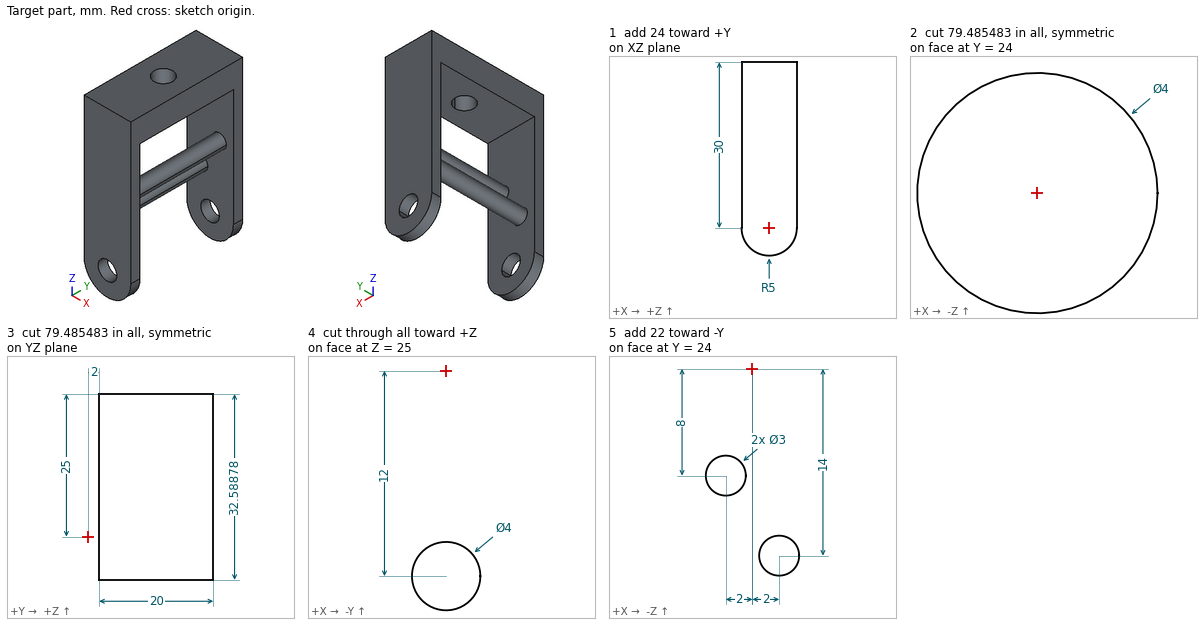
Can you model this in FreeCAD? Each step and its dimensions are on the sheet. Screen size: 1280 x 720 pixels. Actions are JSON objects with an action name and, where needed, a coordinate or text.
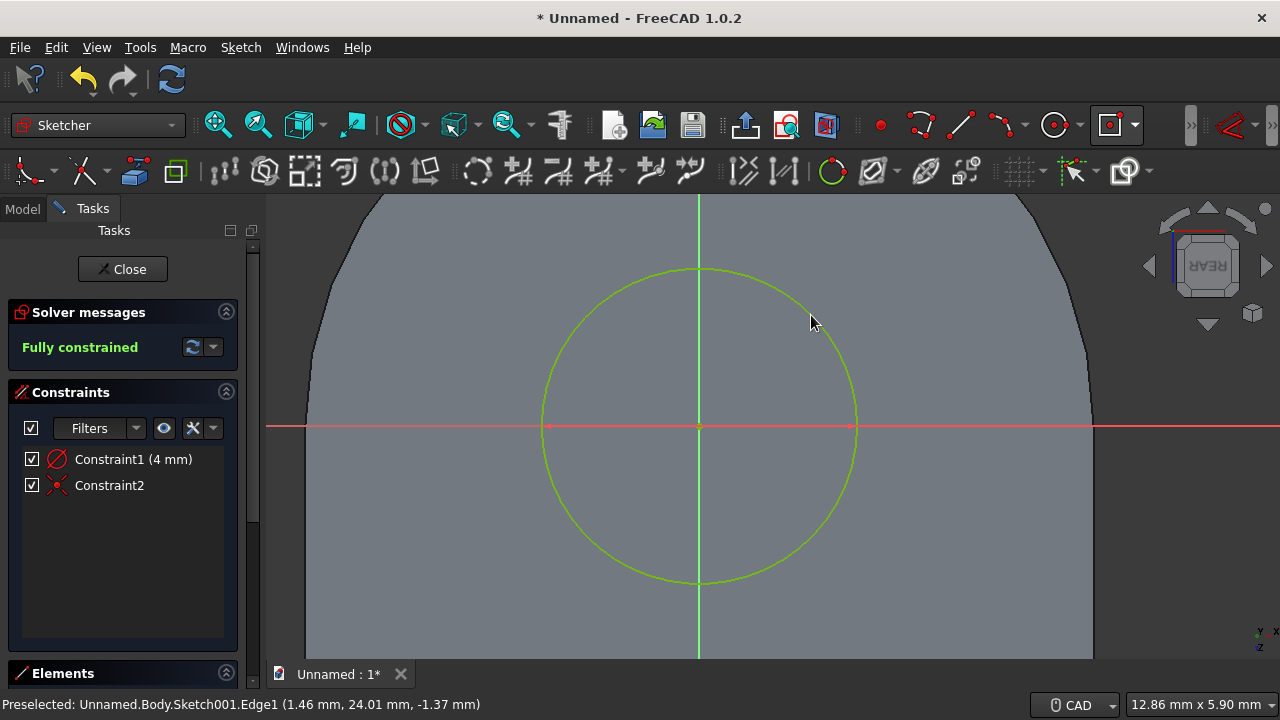
{"action": "left_click", "coordinate": [123, 269]}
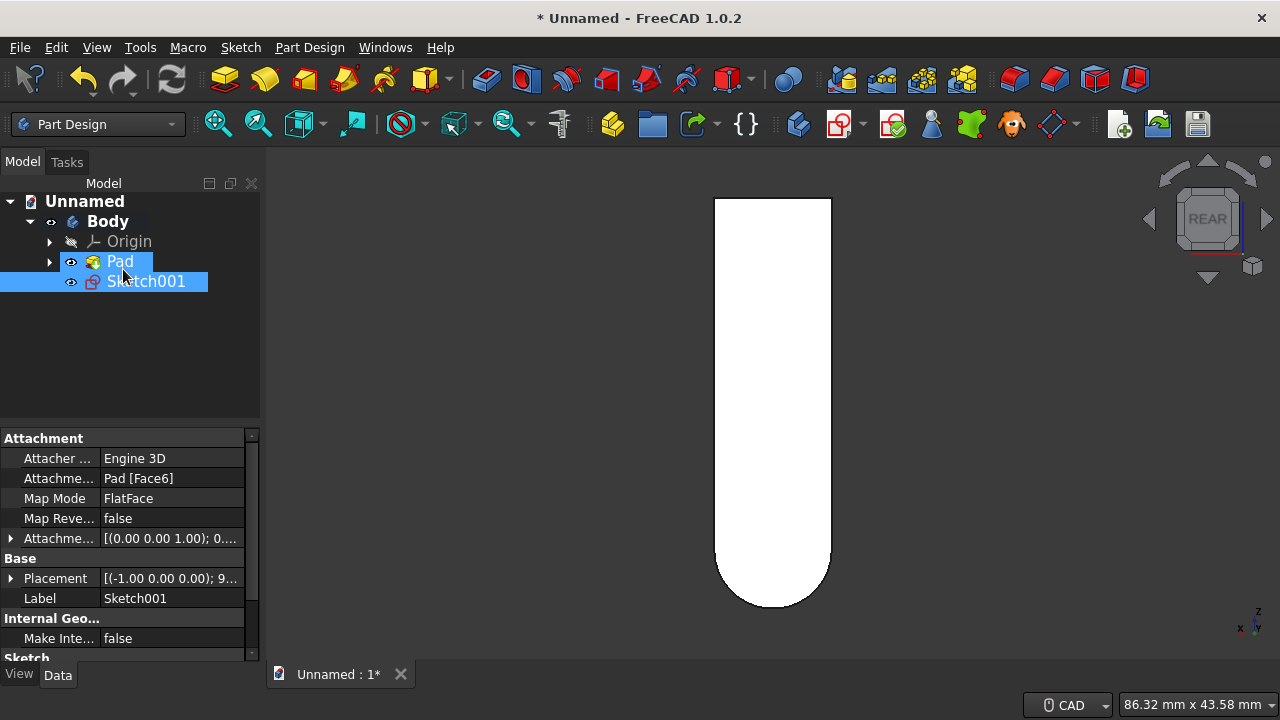
{"action": "left_click", "coordinate": [488, 80]}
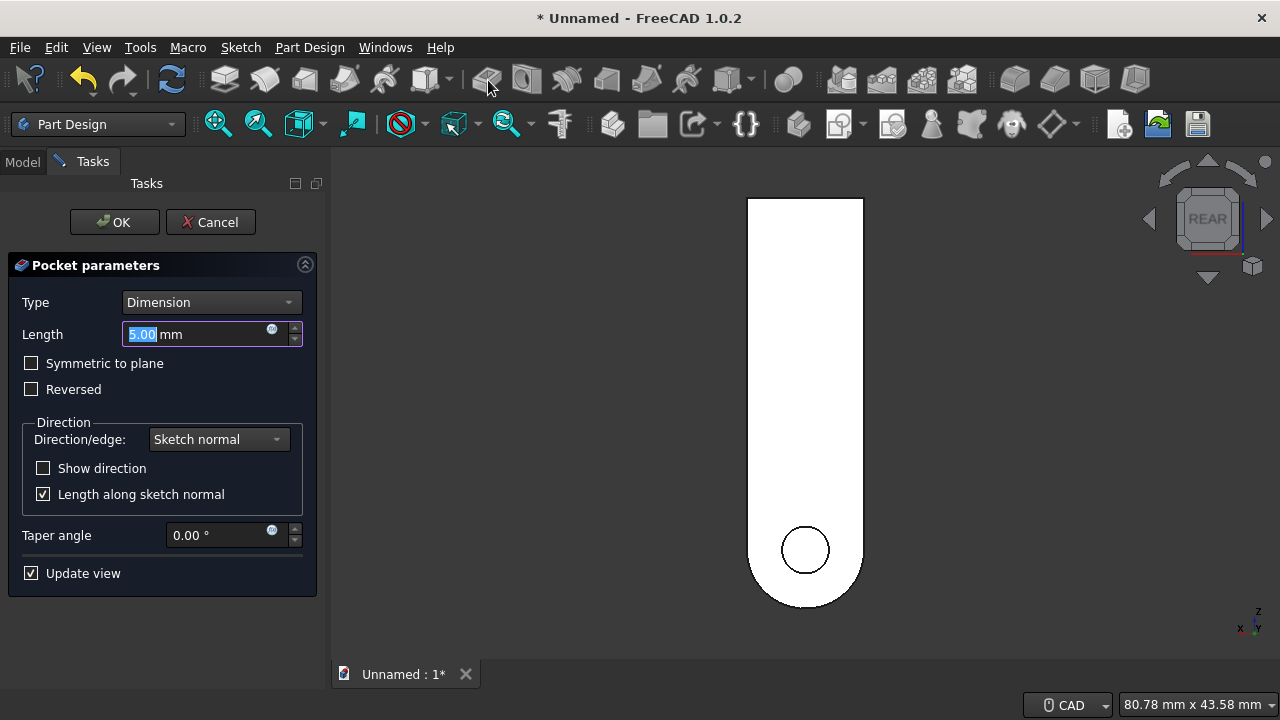
{"action": "type", "text": "79.485483"}
{"action": "key", "text": "Tab"}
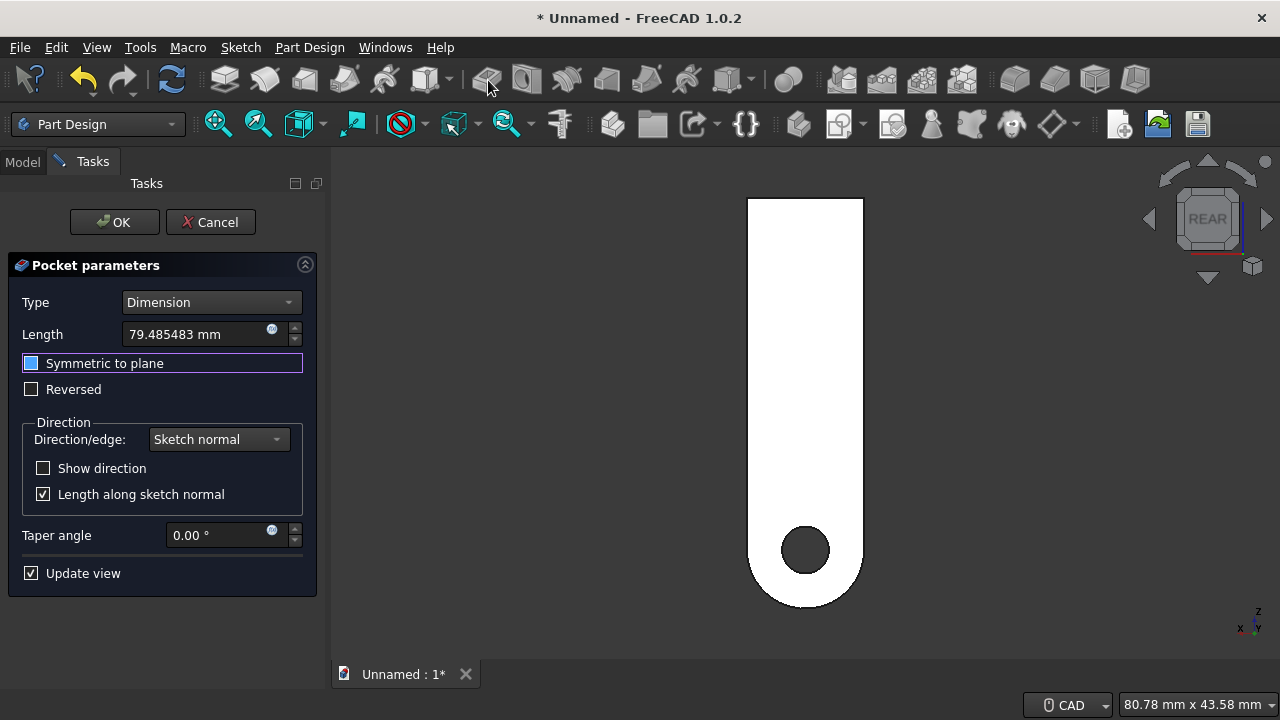
{"action": "left_click", "coordinate": [30, 363]}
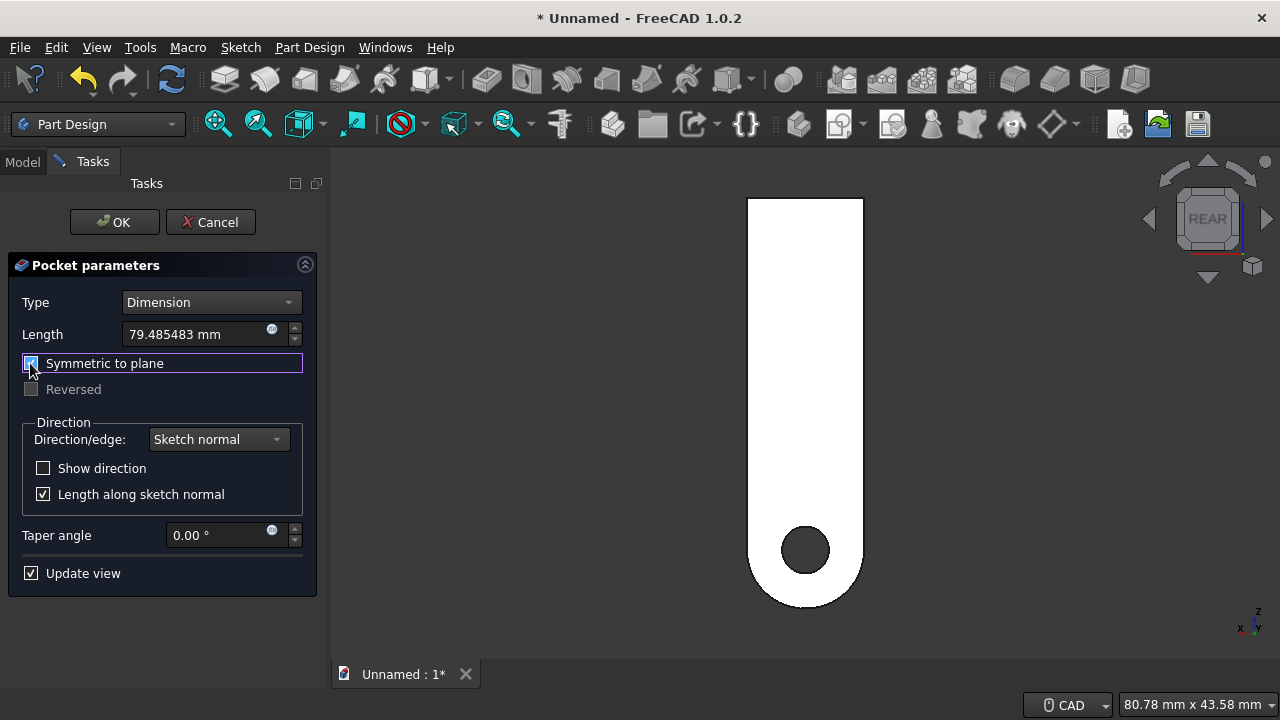
{"action": "left_click", "coordinate": [115, 222]}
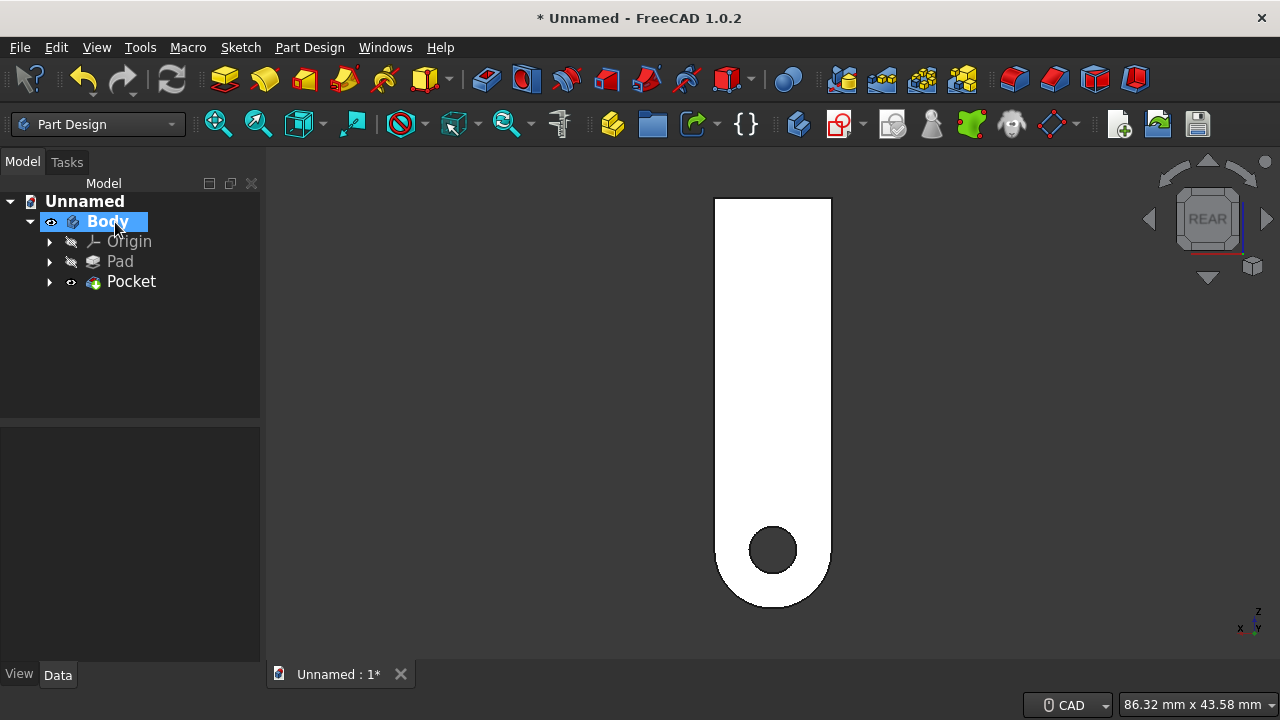
{"action": "left_click", "coordinate": [840, 124]}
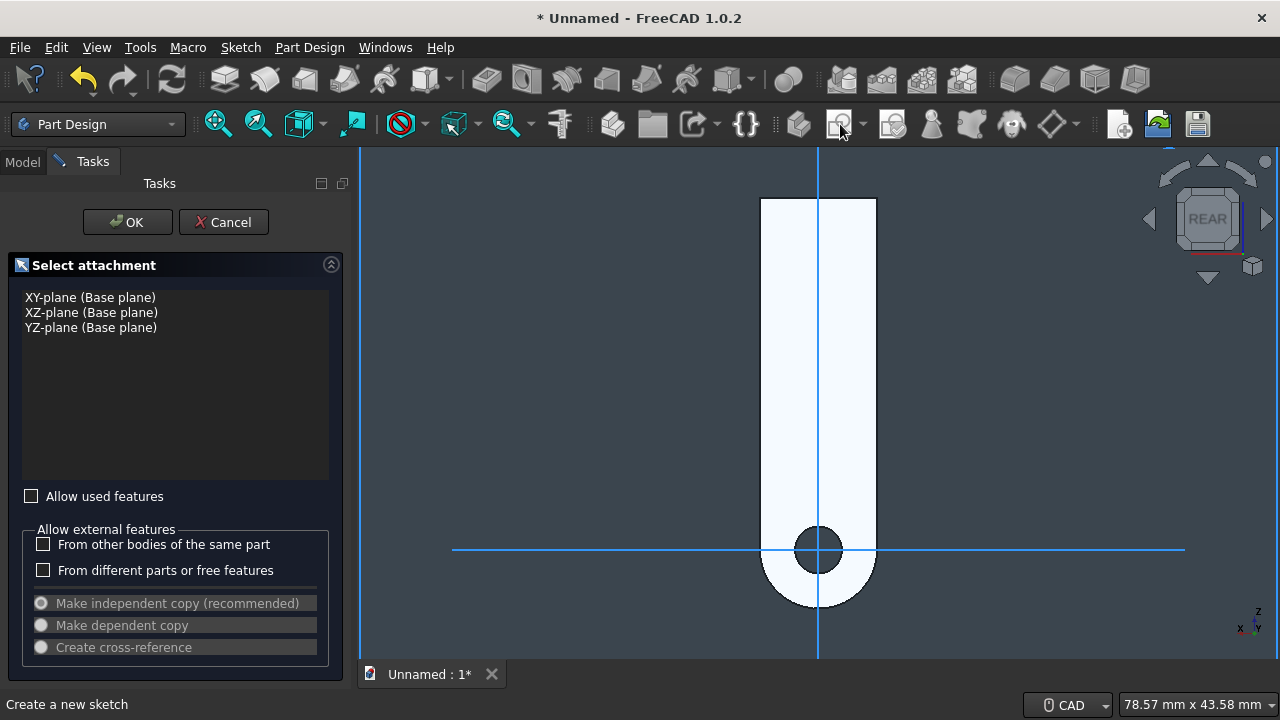
{"action": "left_click", "coordinate": [82, 328]}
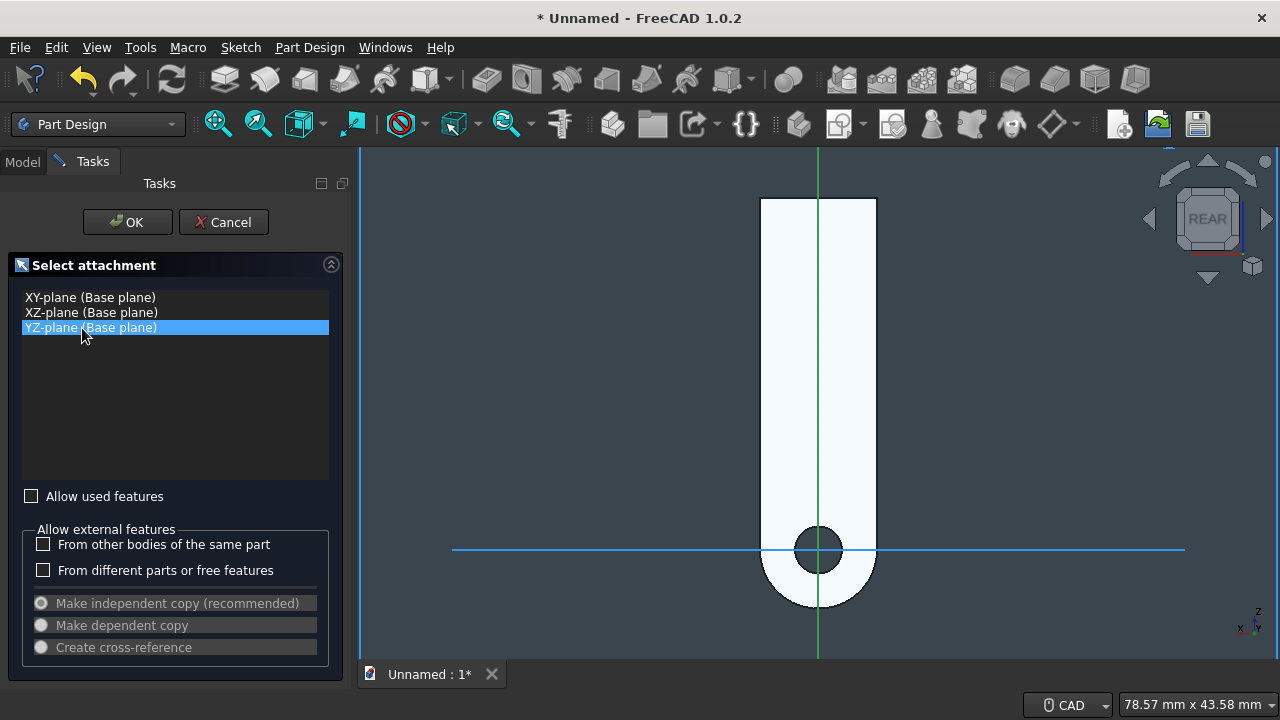
{"action": "left_click", "coordinate": [128, 222]}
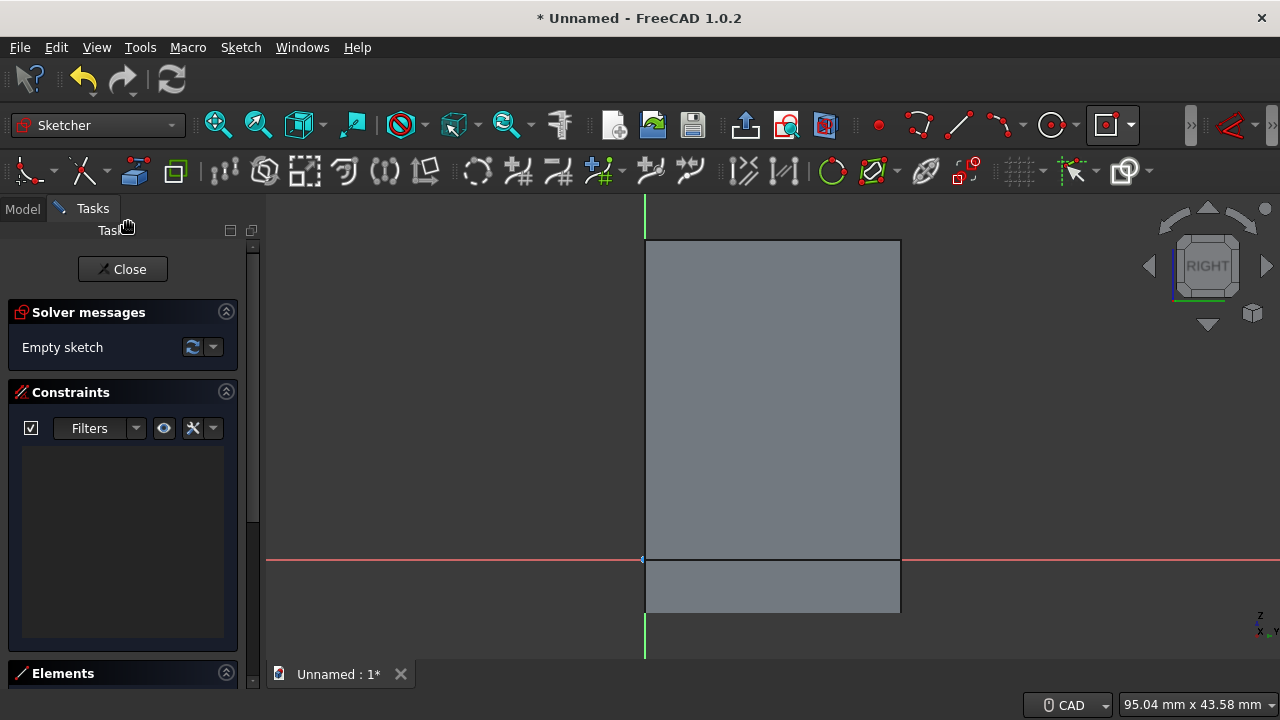
{"action": "left_click", "coordinate": [826, 126]}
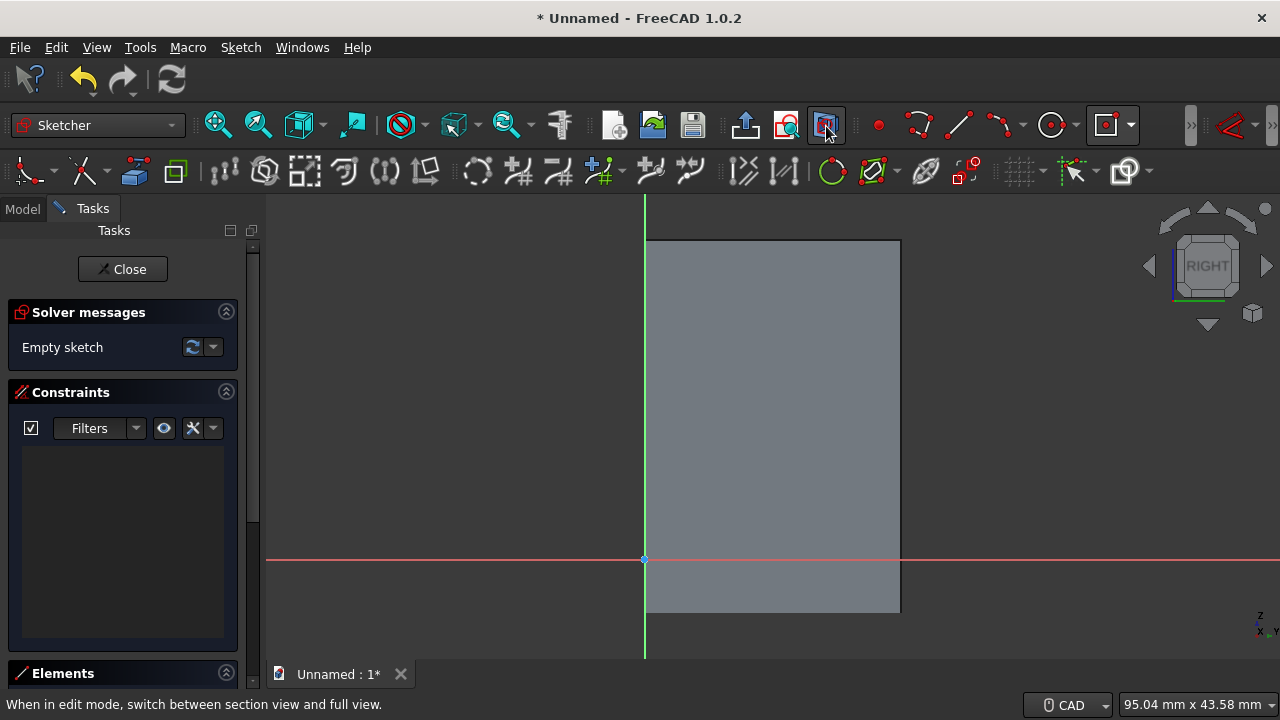
{"action": "scroll", "coordinate": [443, 243], "scroll_direction": "down", "scroll_amount": 1}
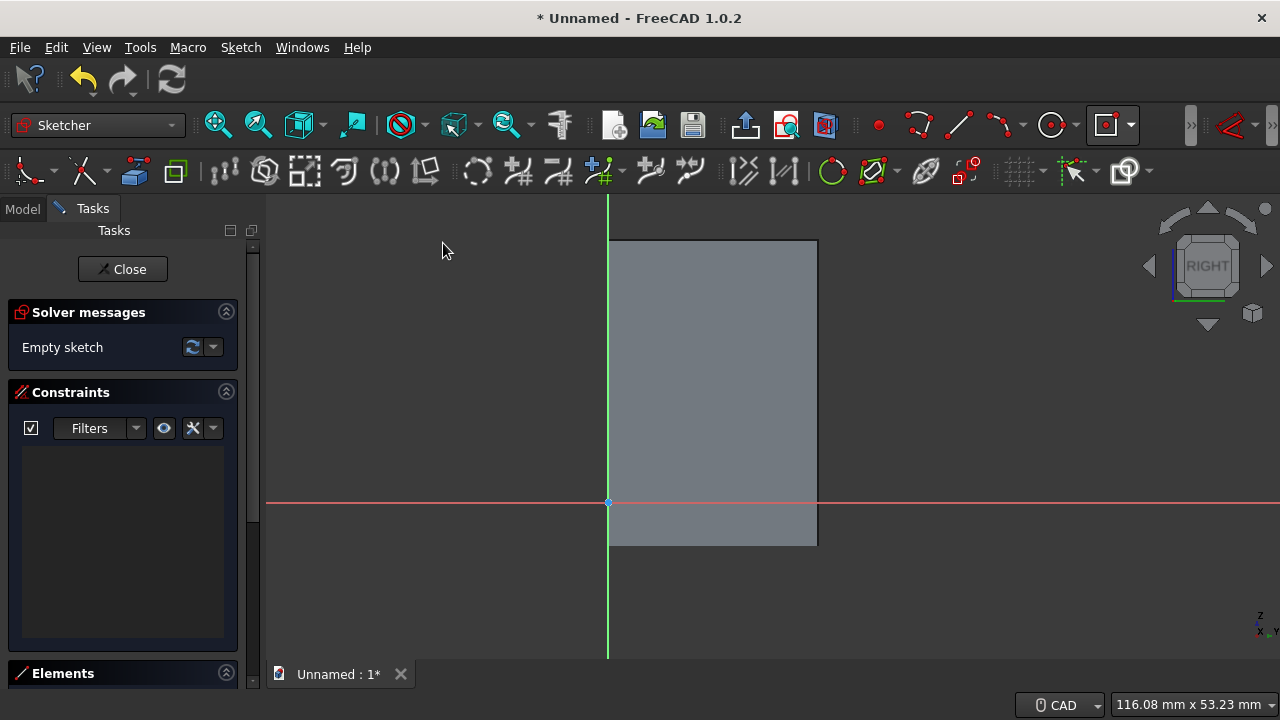
{"action": "left_click", "coordinate": [1134, 126]}